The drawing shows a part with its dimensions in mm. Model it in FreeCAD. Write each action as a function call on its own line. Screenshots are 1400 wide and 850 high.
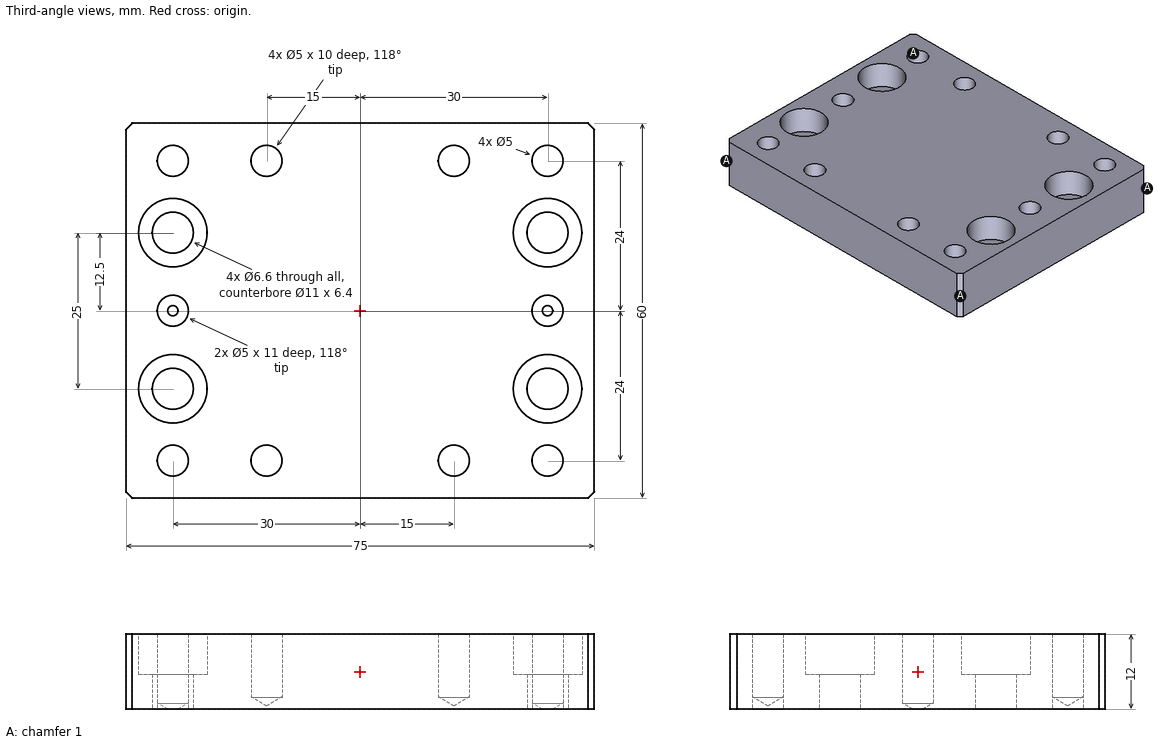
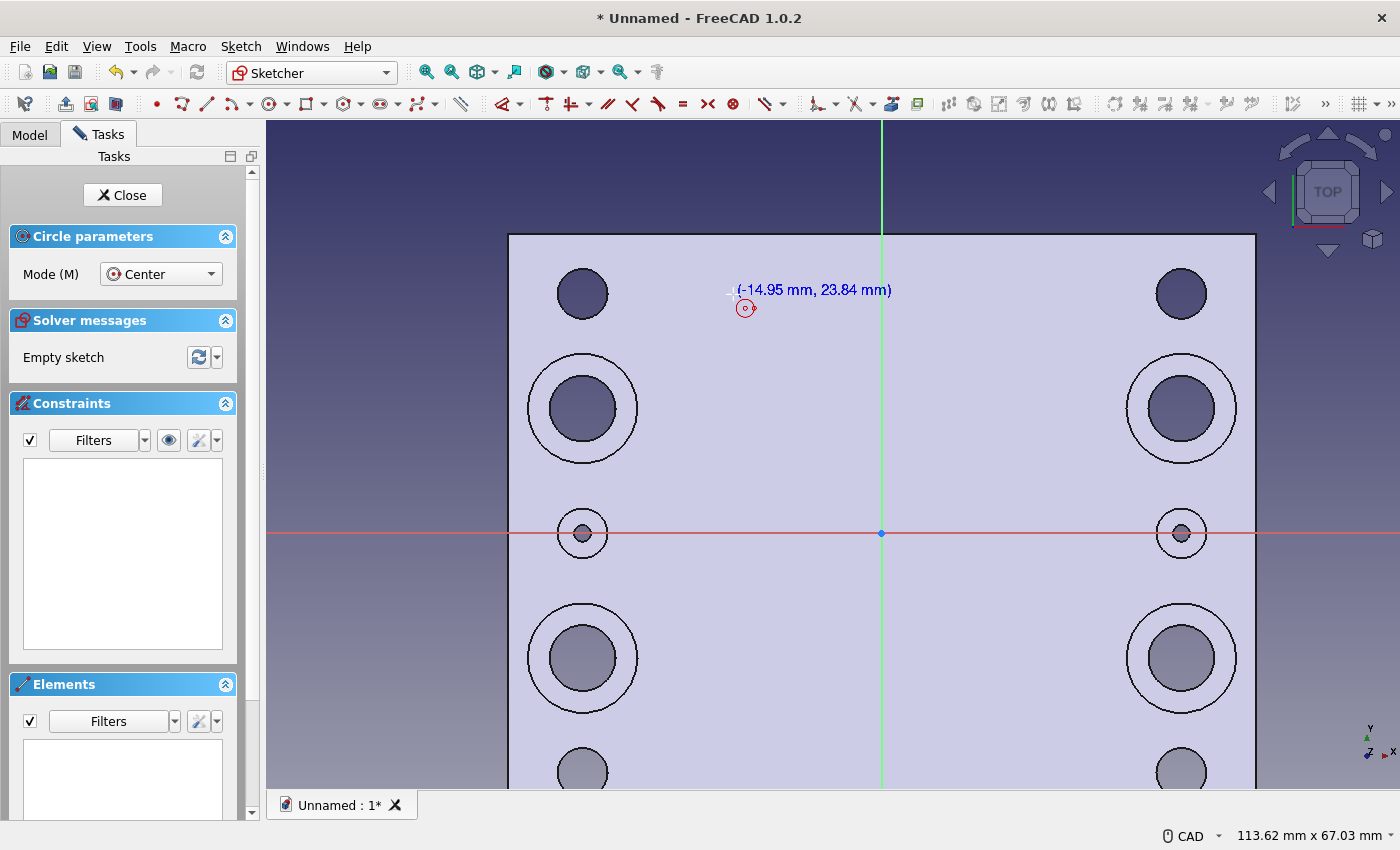
click(732, 294)
click(750, 276)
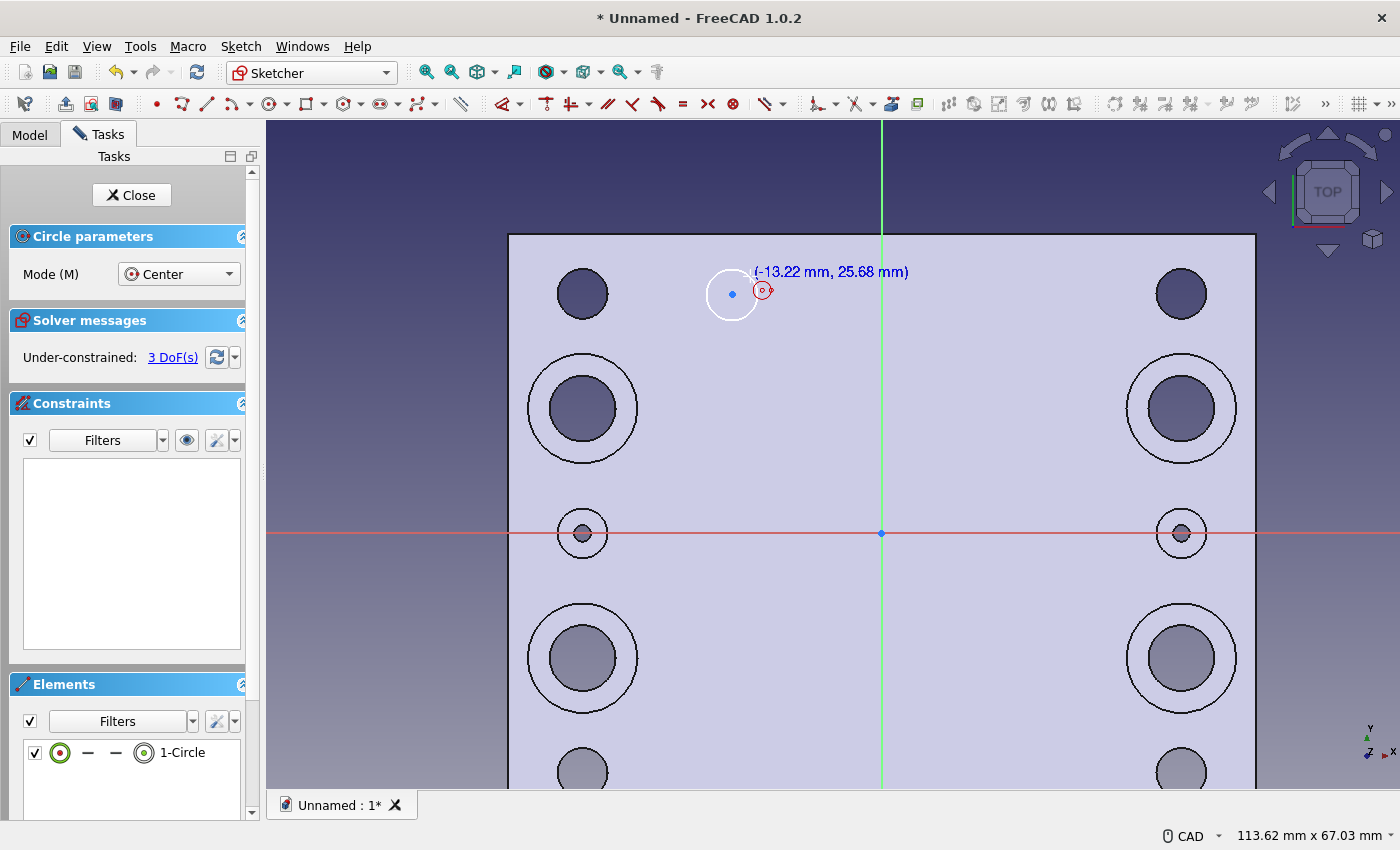
scroll(294, 148, down, 1)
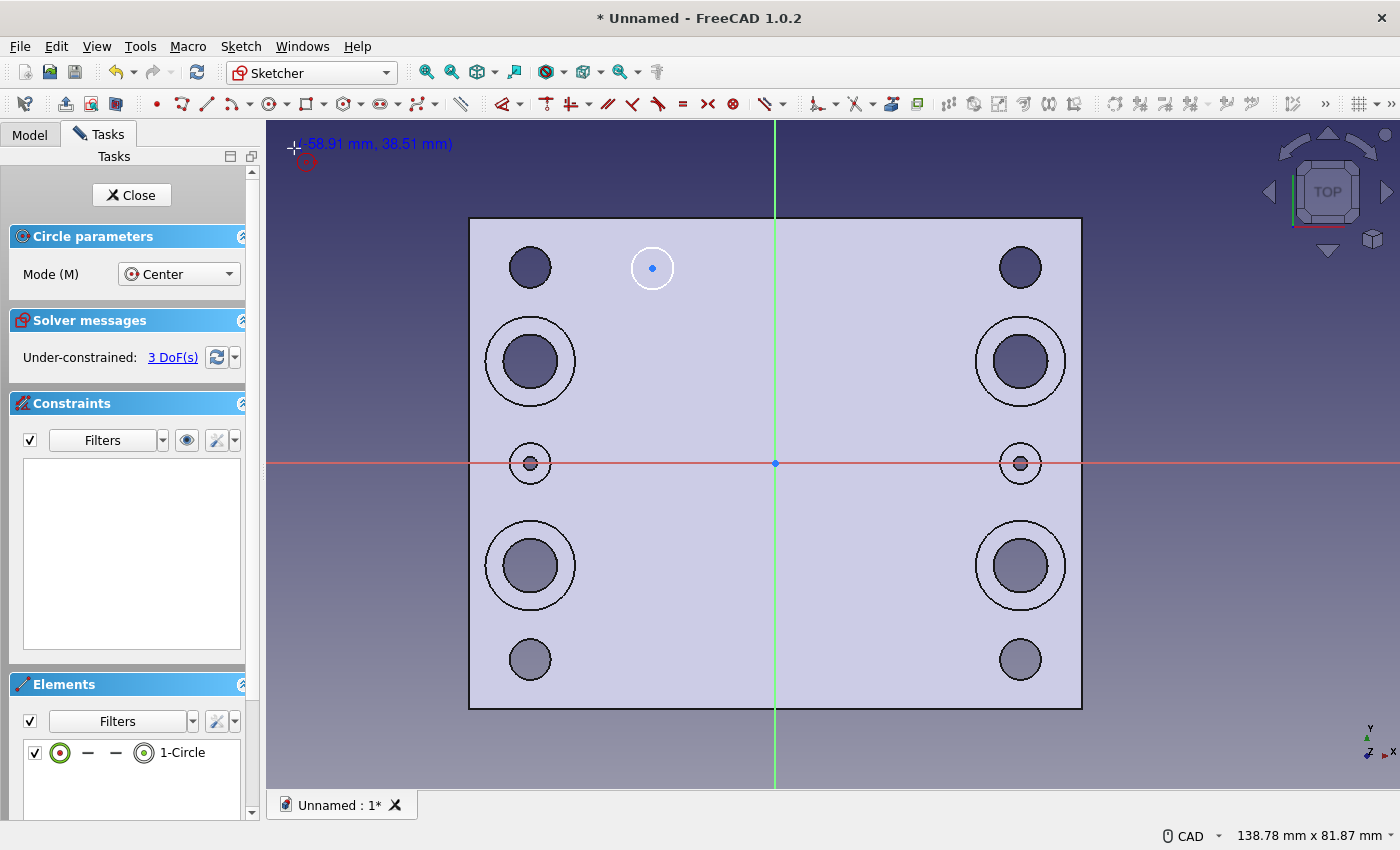
click(898, 660)
click(912, 645)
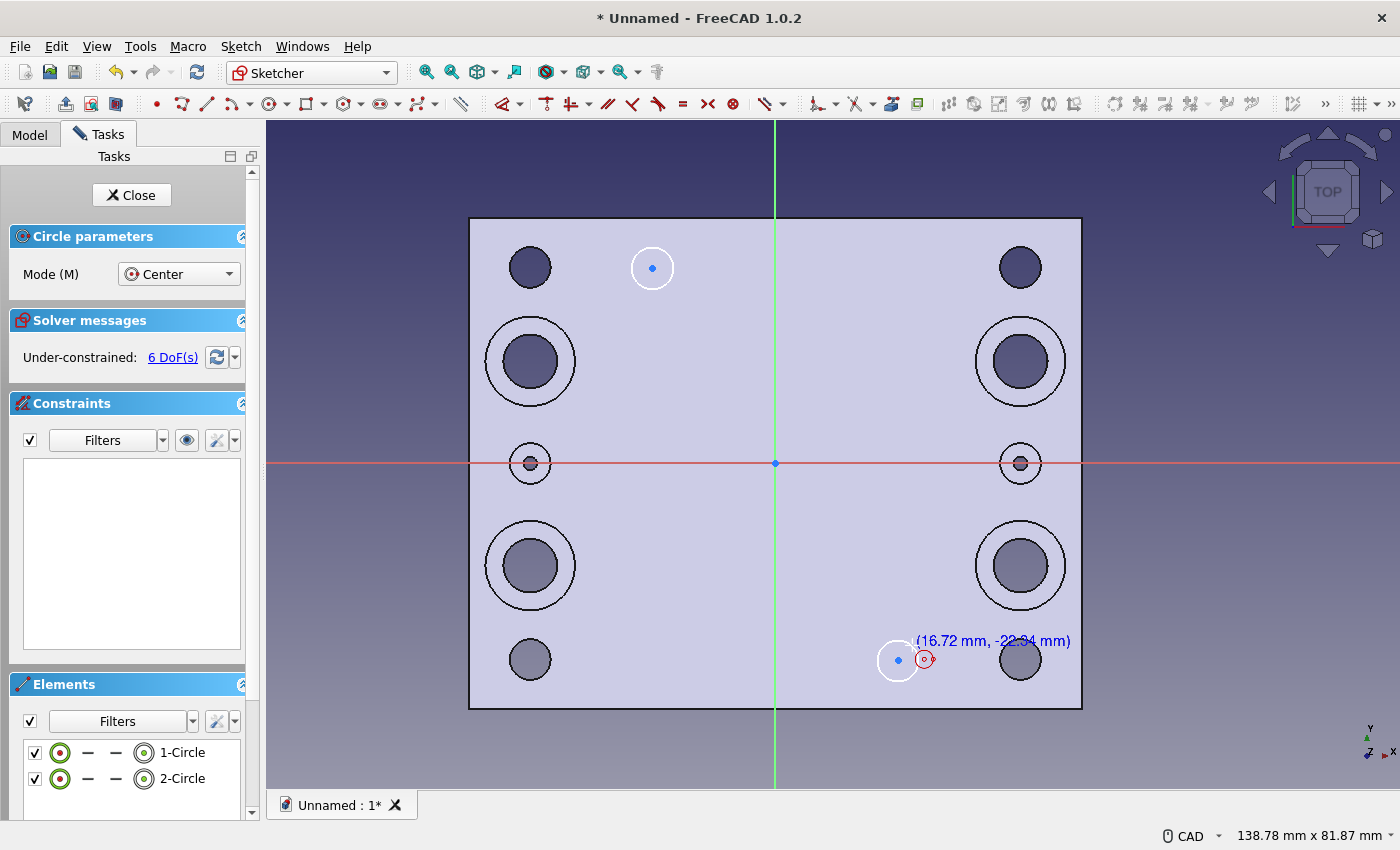
click(898, 267)
click(912, 253)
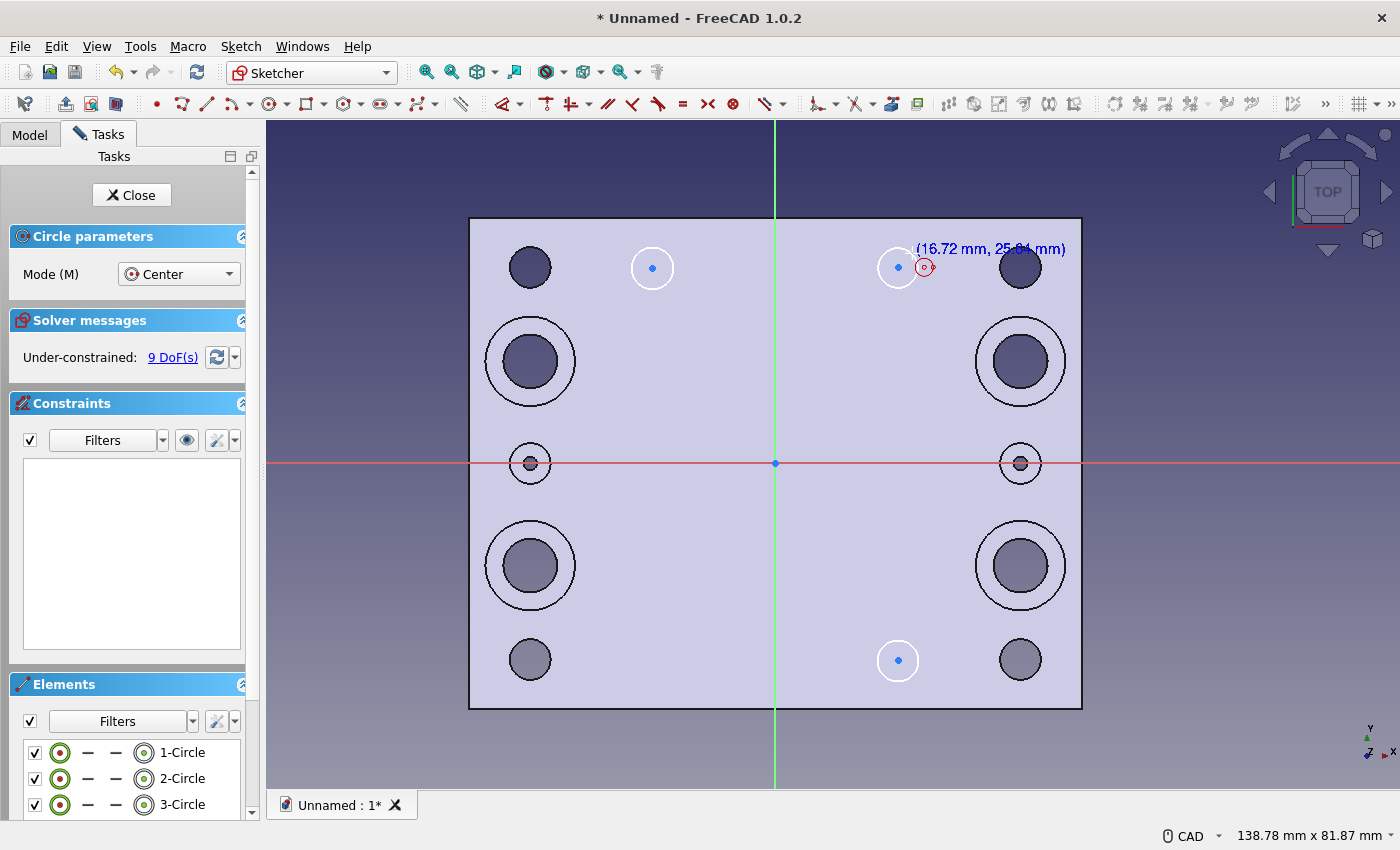
click(653, 660)
click(667, 645)
key(Escape)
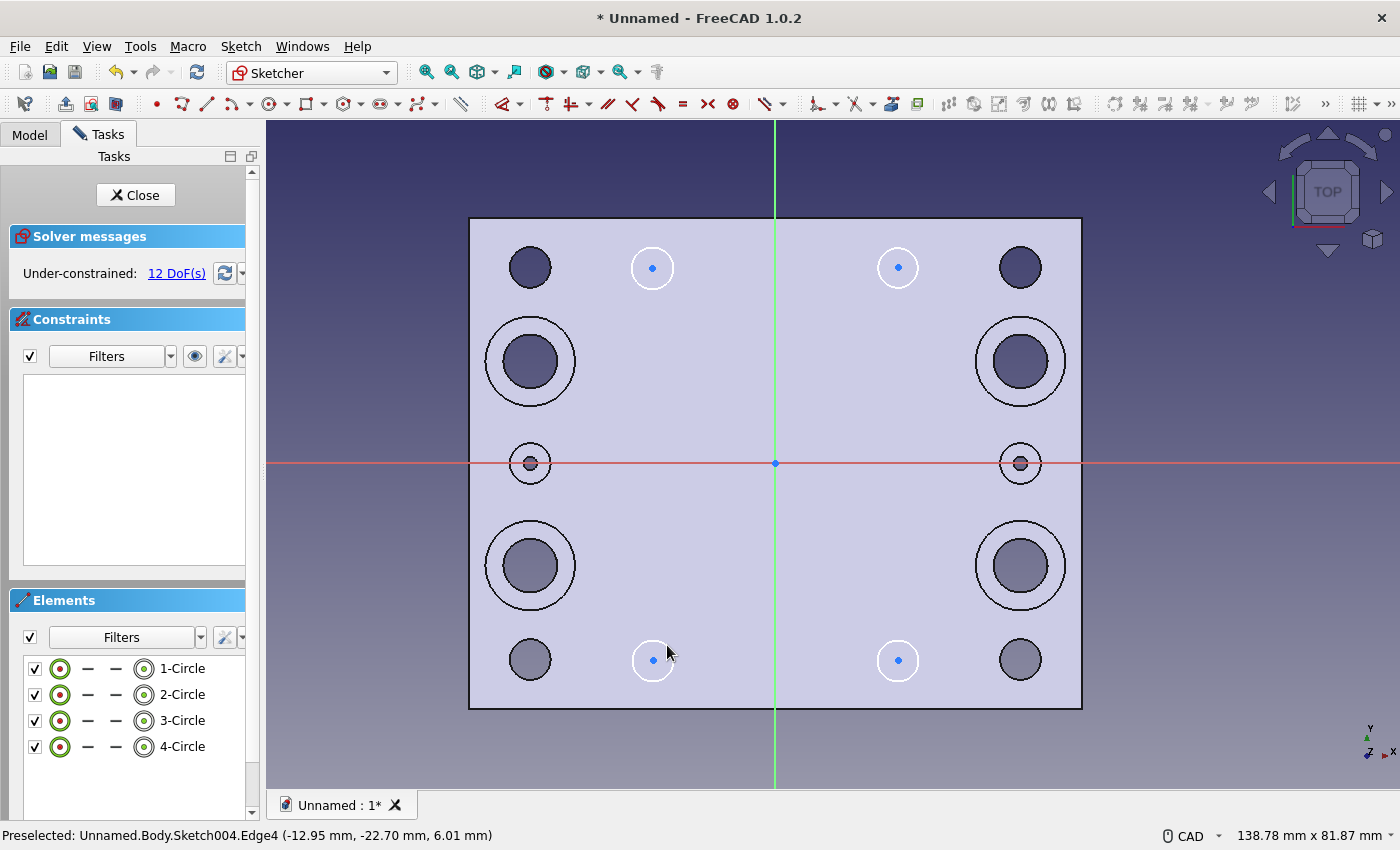
click(667, 254)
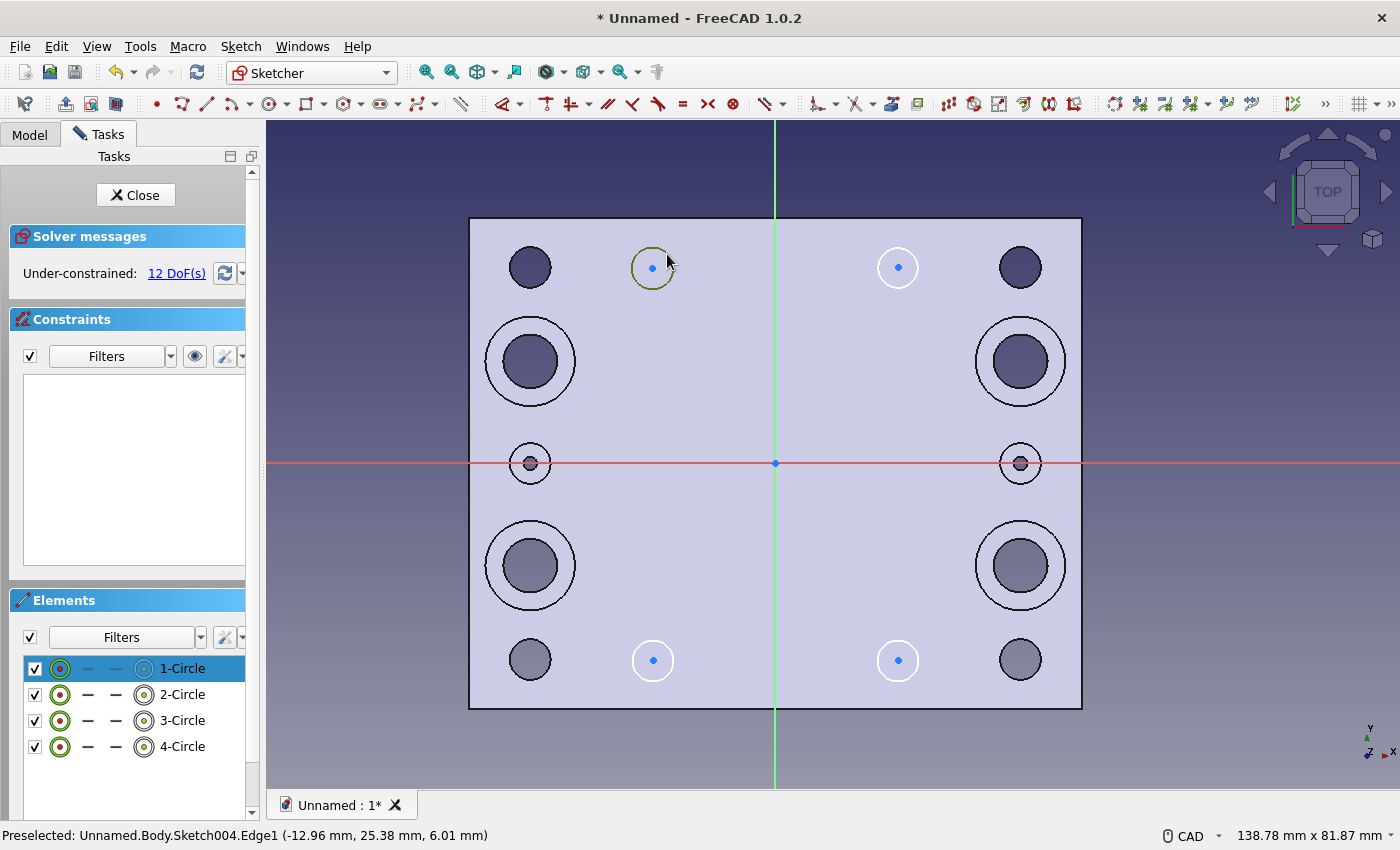
click(912, 646)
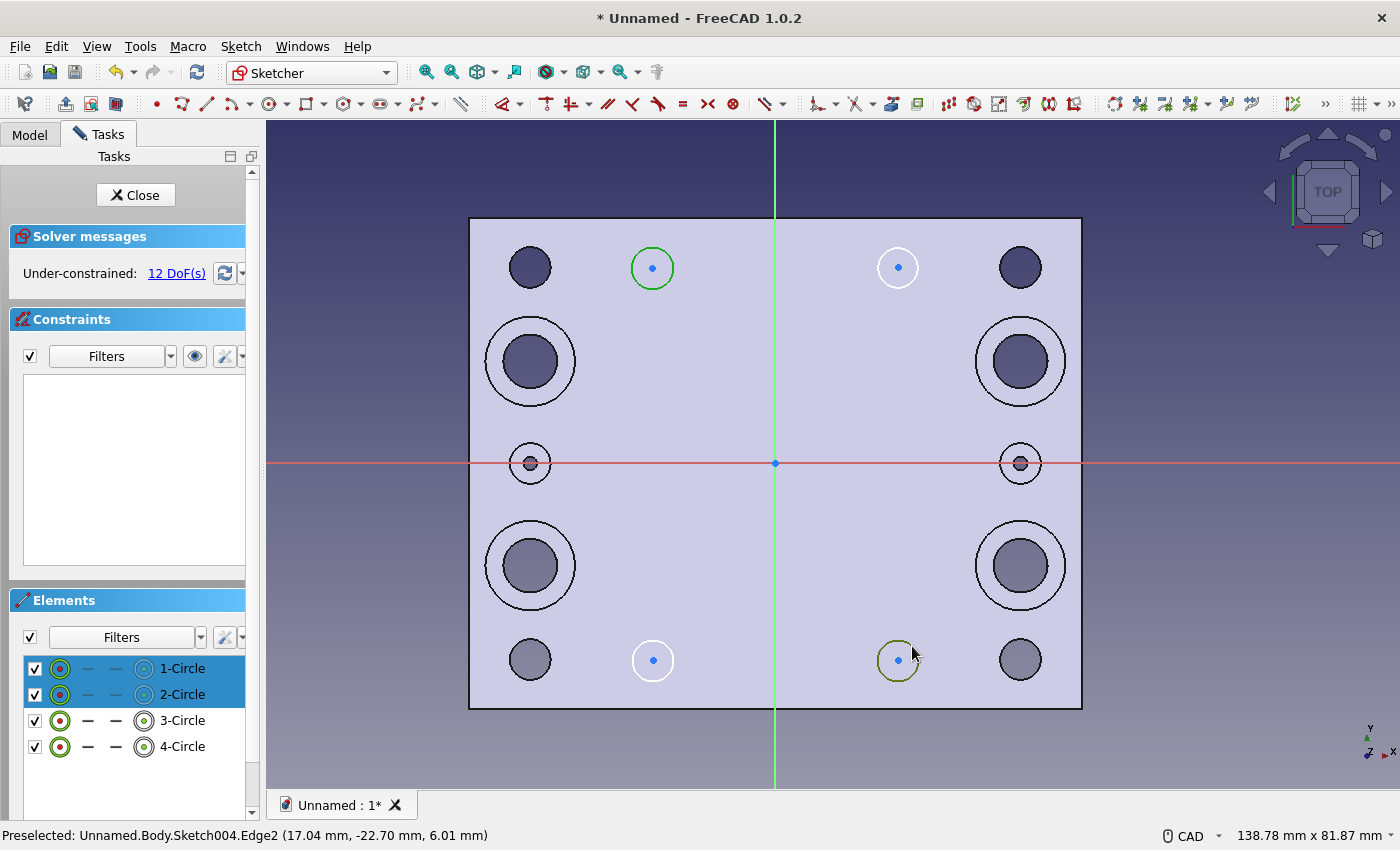
click(912, 254)